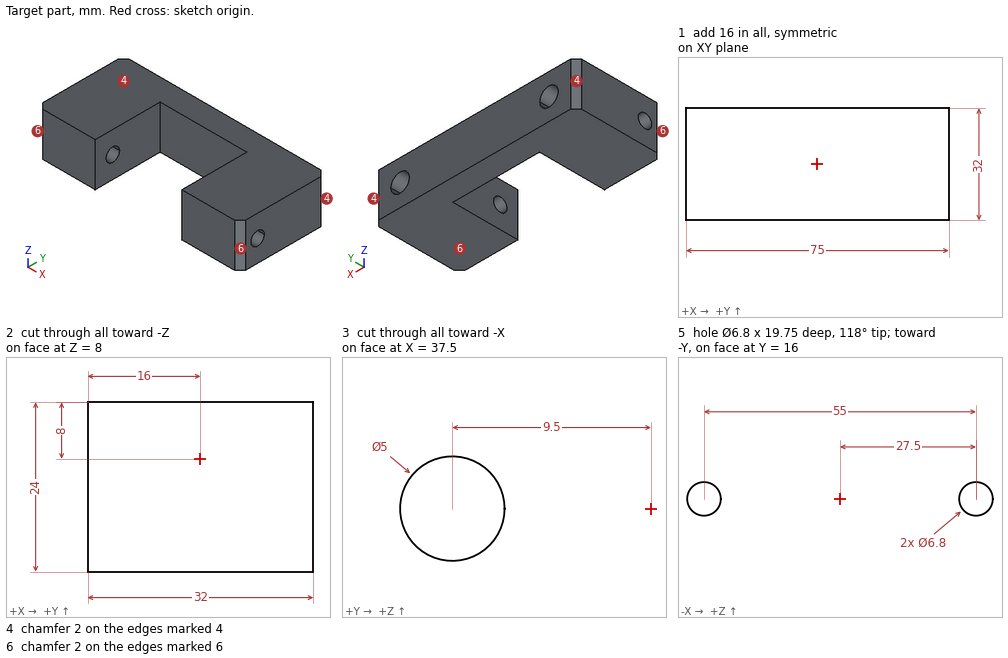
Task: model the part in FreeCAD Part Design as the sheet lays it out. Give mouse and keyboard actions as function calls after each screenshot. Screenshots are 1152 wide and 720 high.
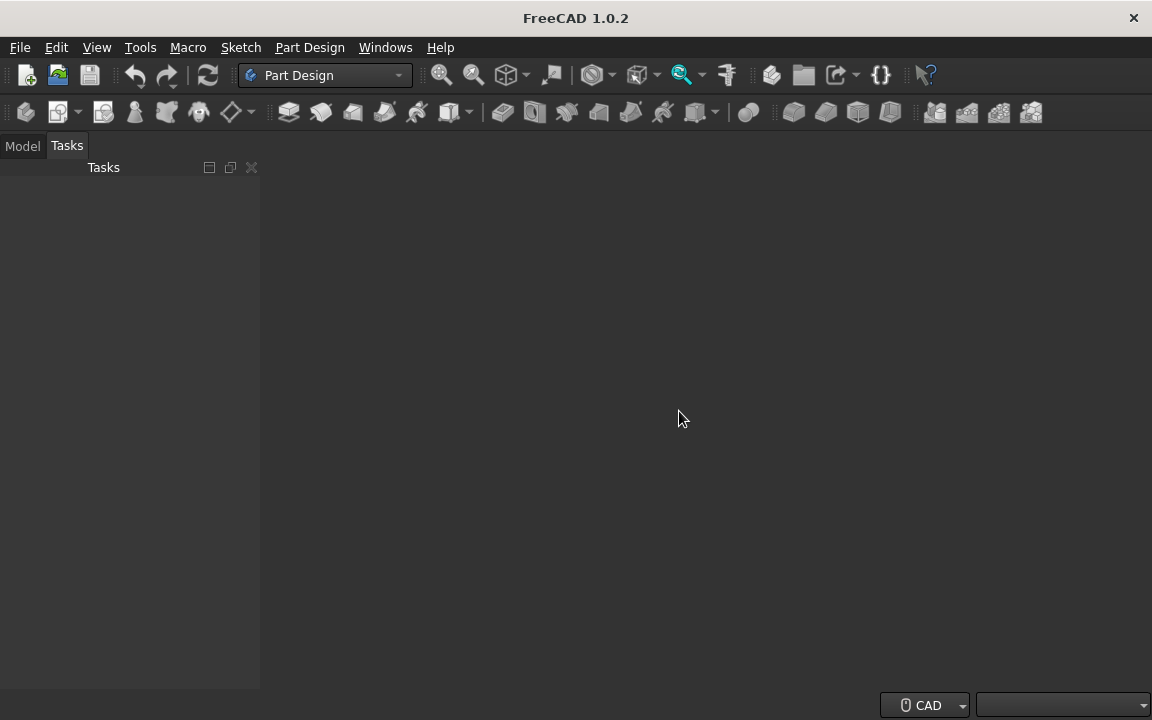
key(ctrl+n)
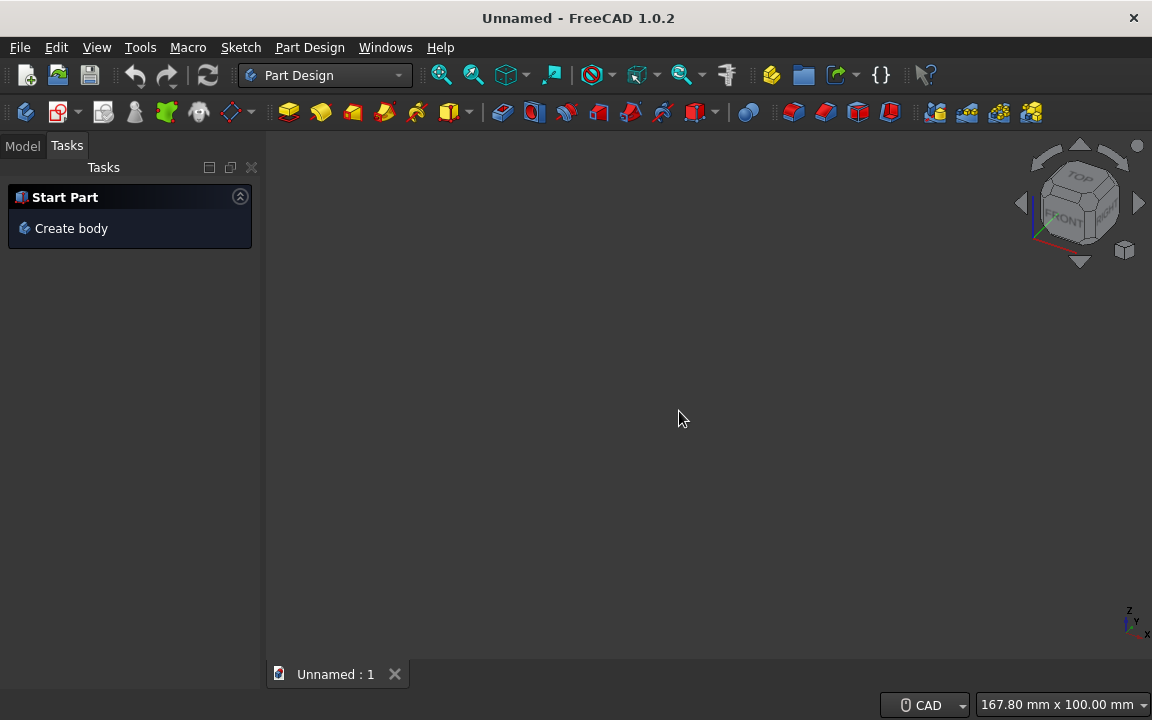
click(58, 112)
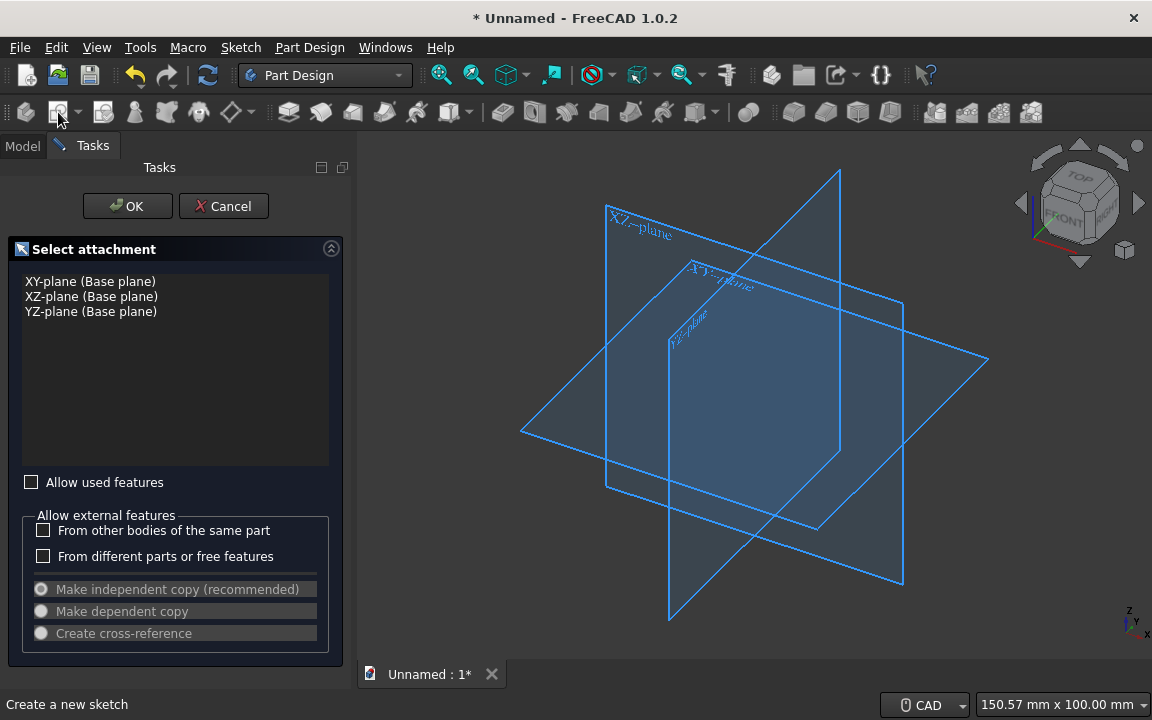
click(82, 282)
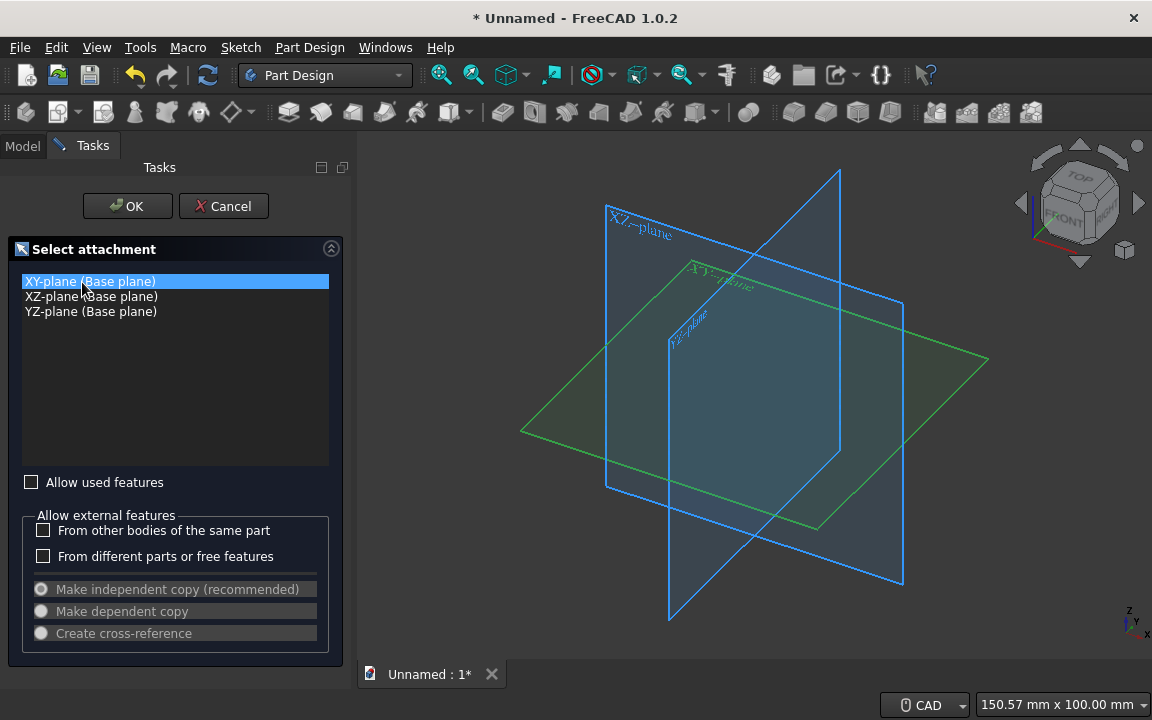
click(128, 206)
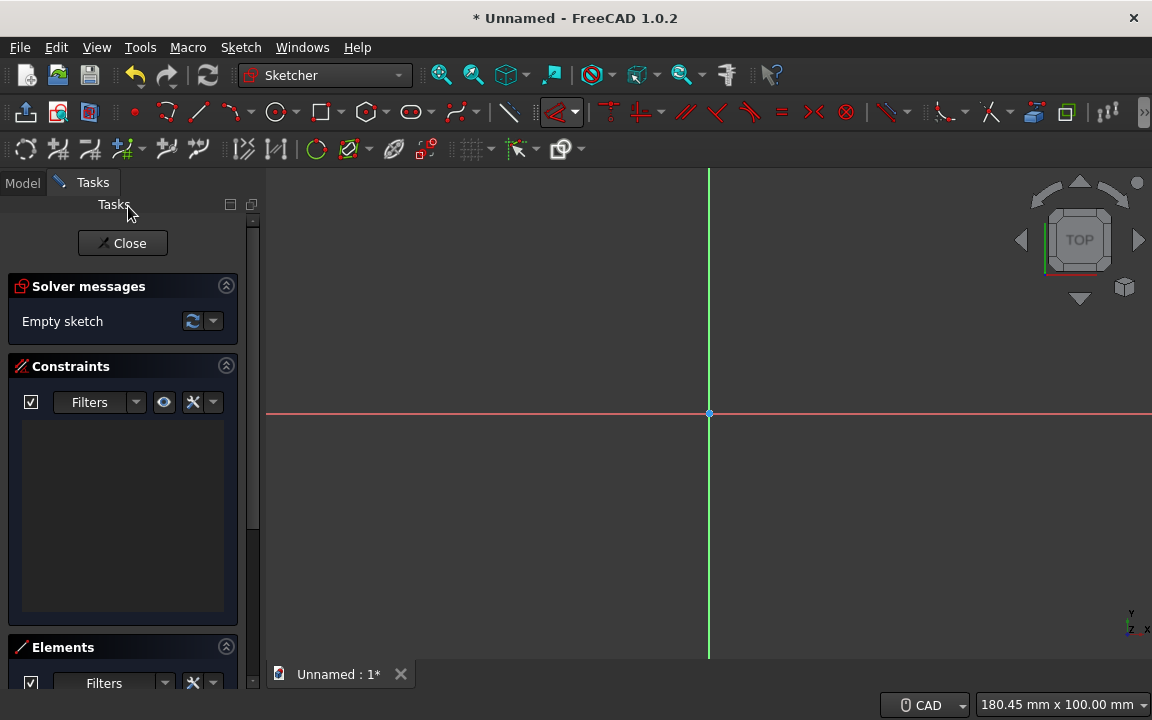
key(g)
key(v)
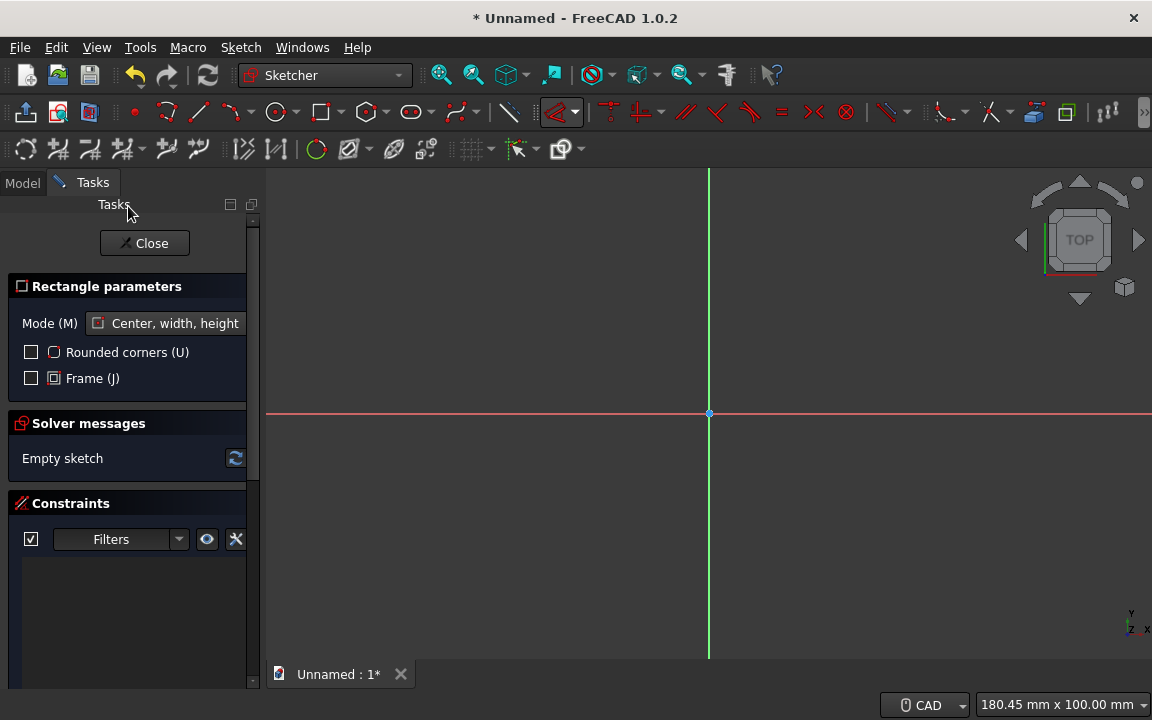
click(709, 414)
click(893, 335)
key(Escape)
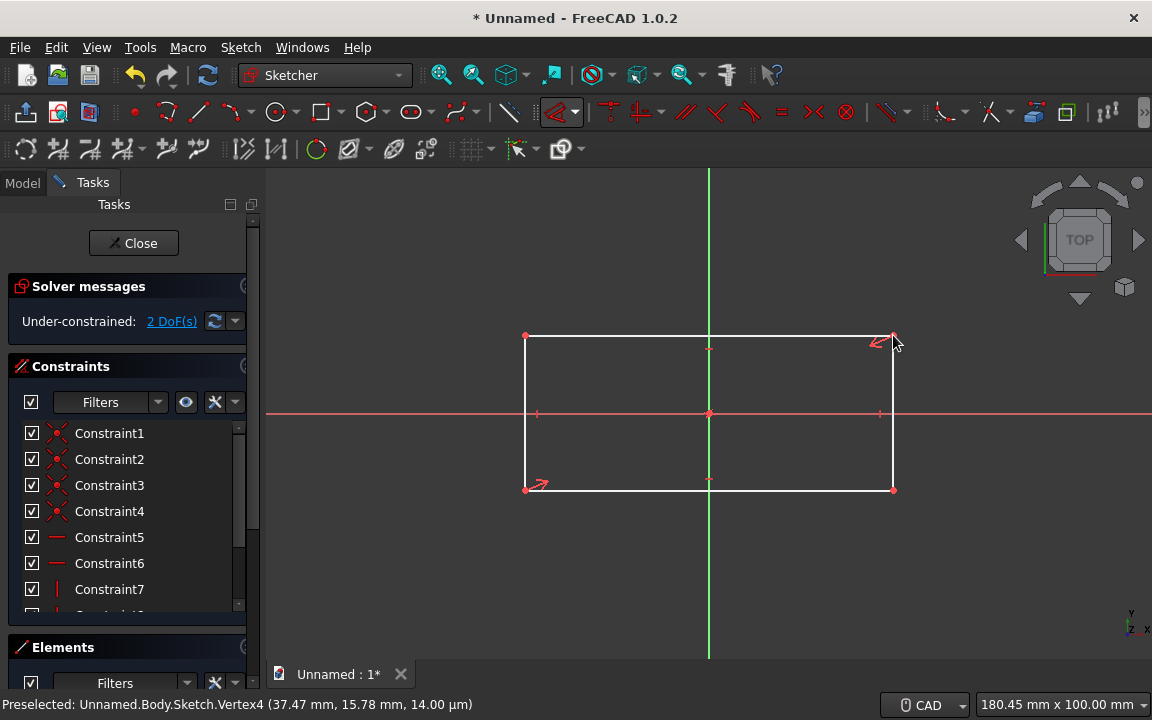
click(635, 491)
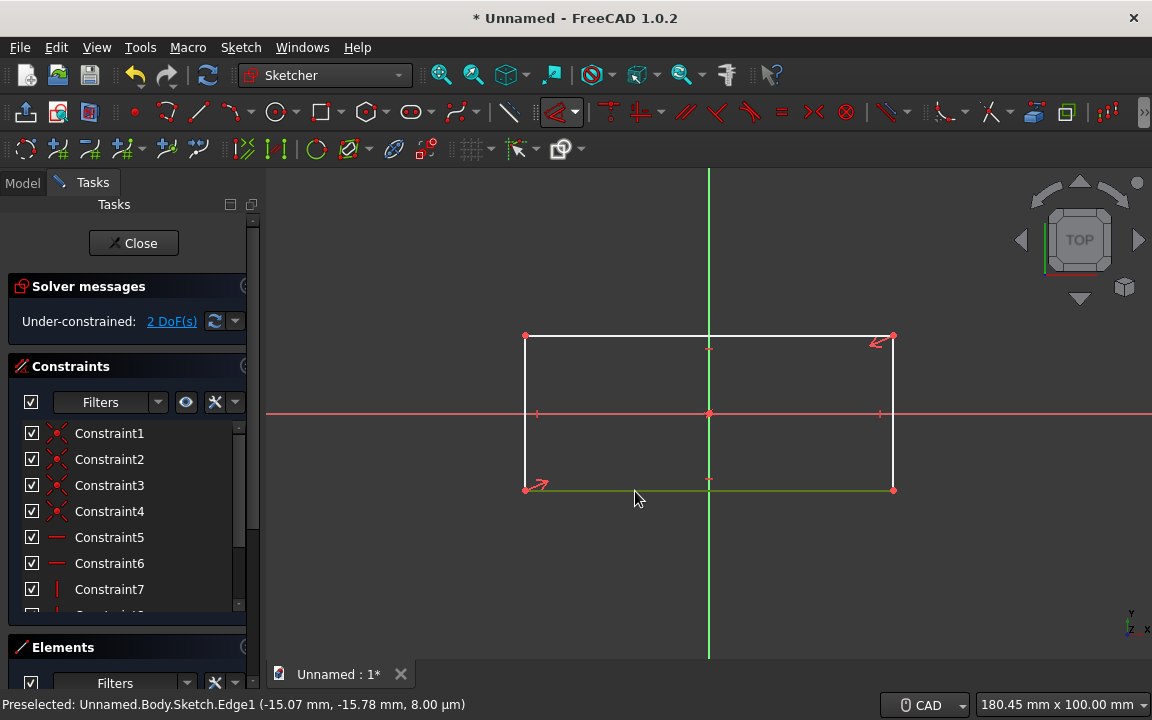
click(578, 112)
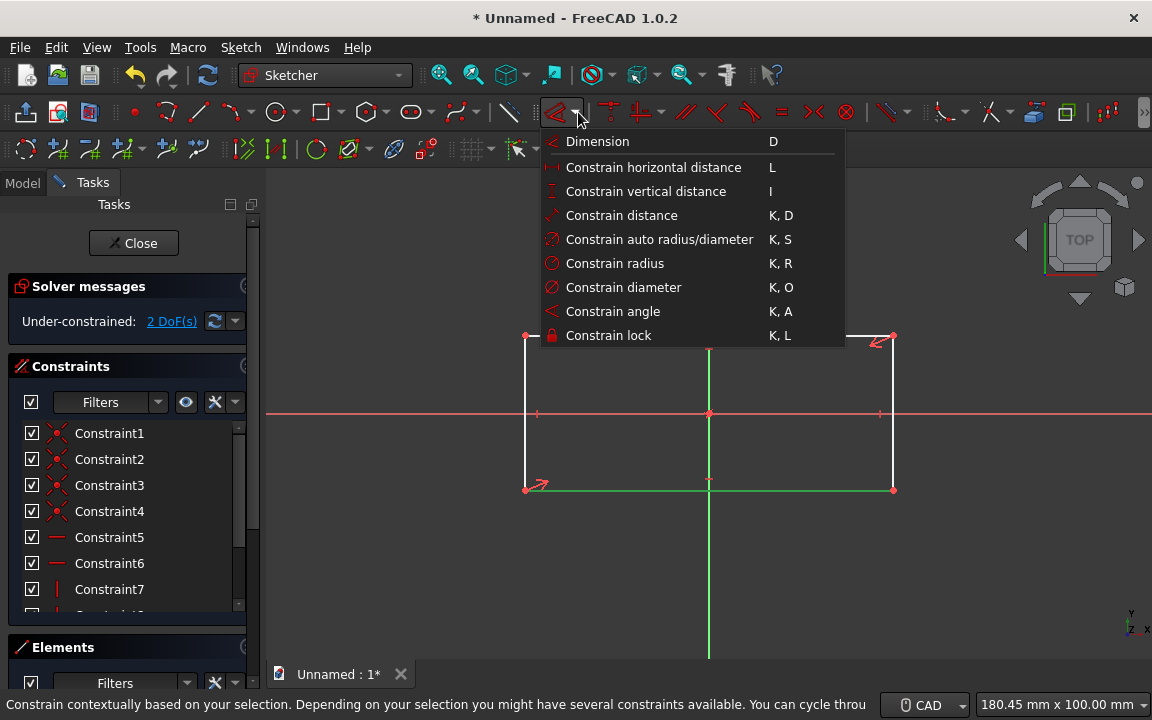
click(693, 167)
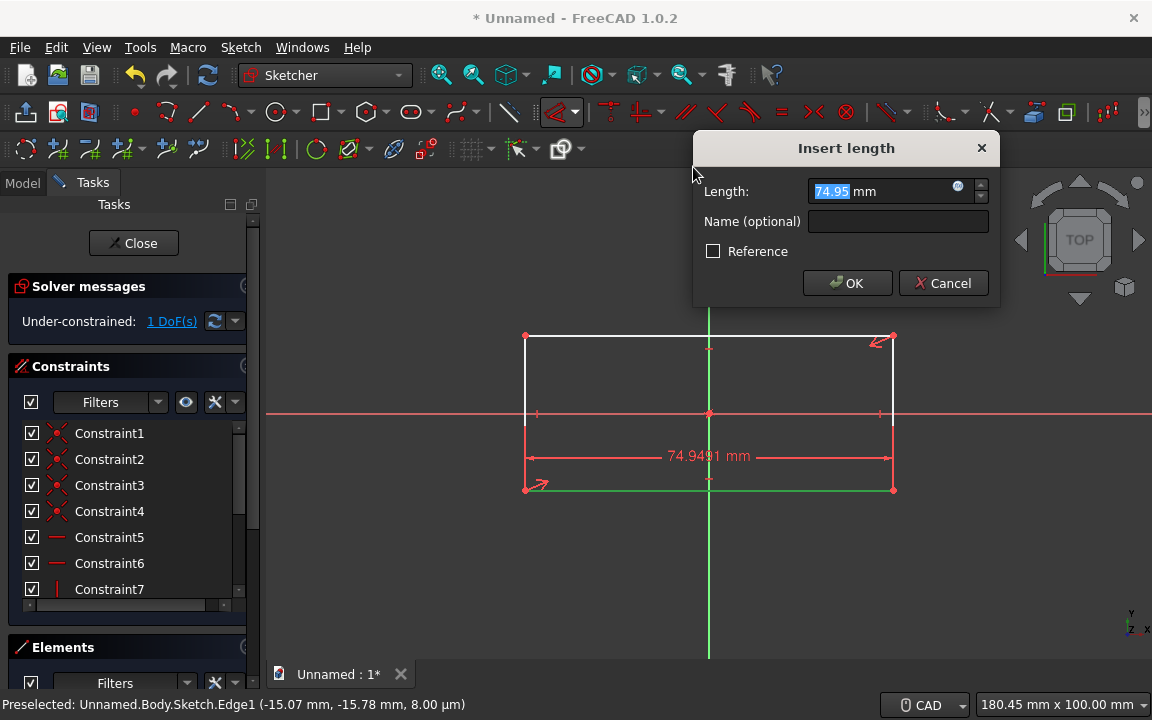
text(75)
key(Return)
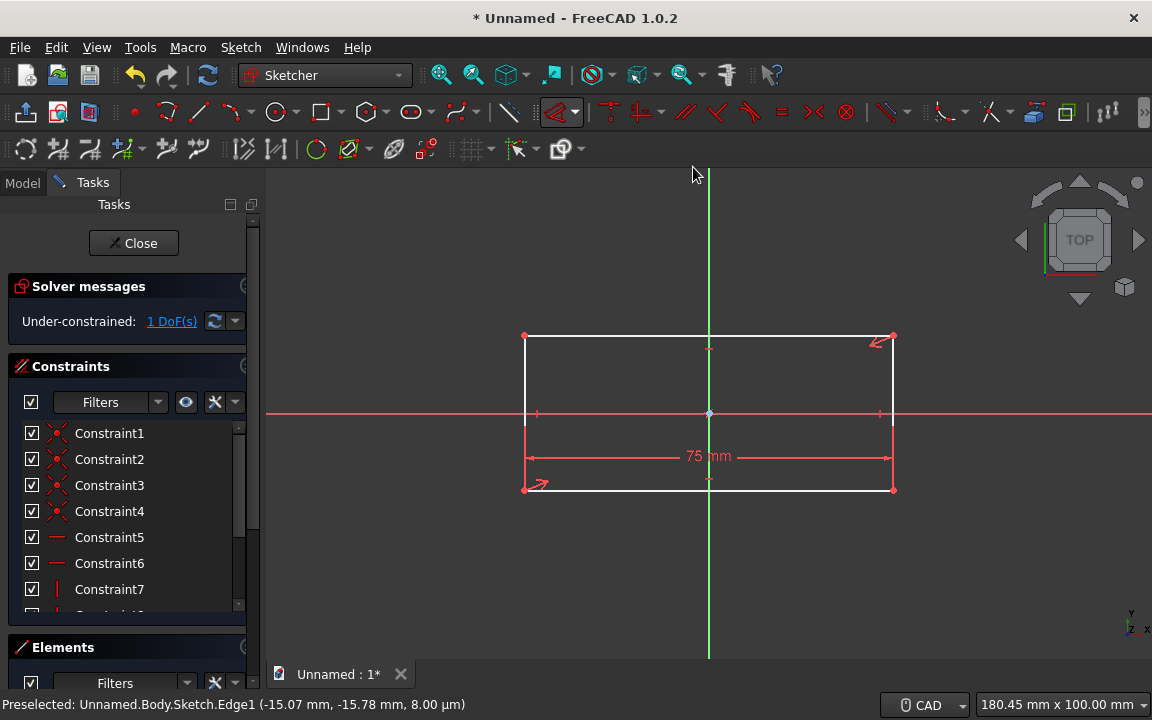
click(893, 445)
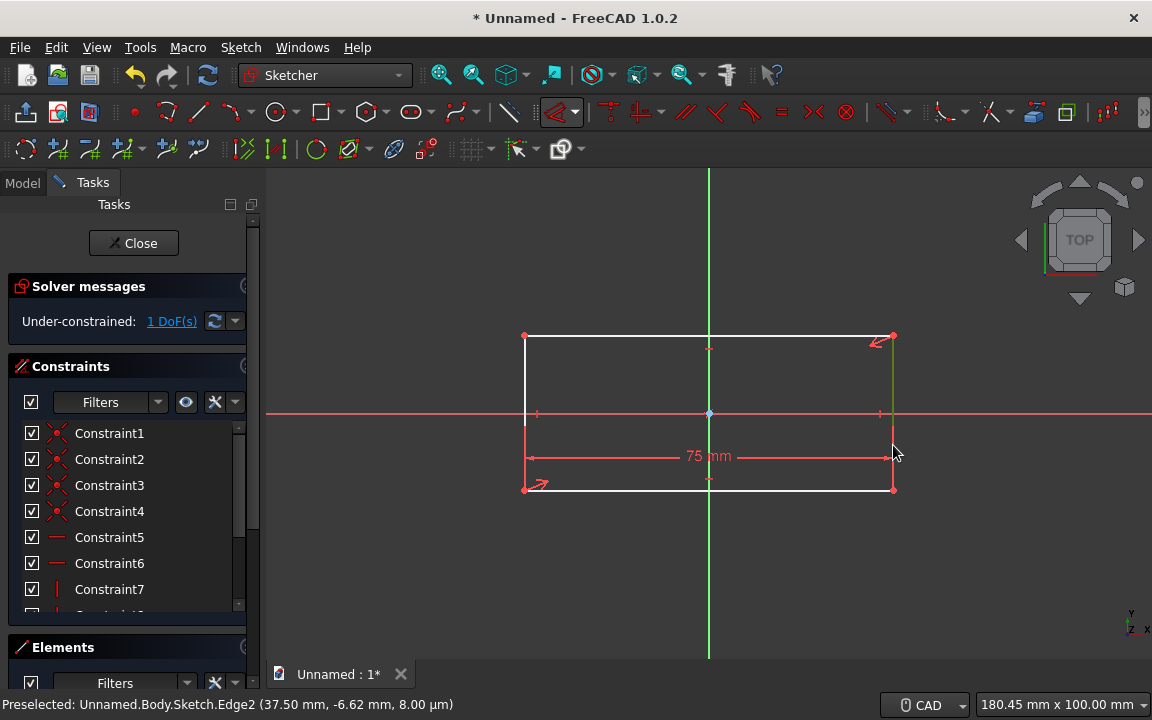
key(i)